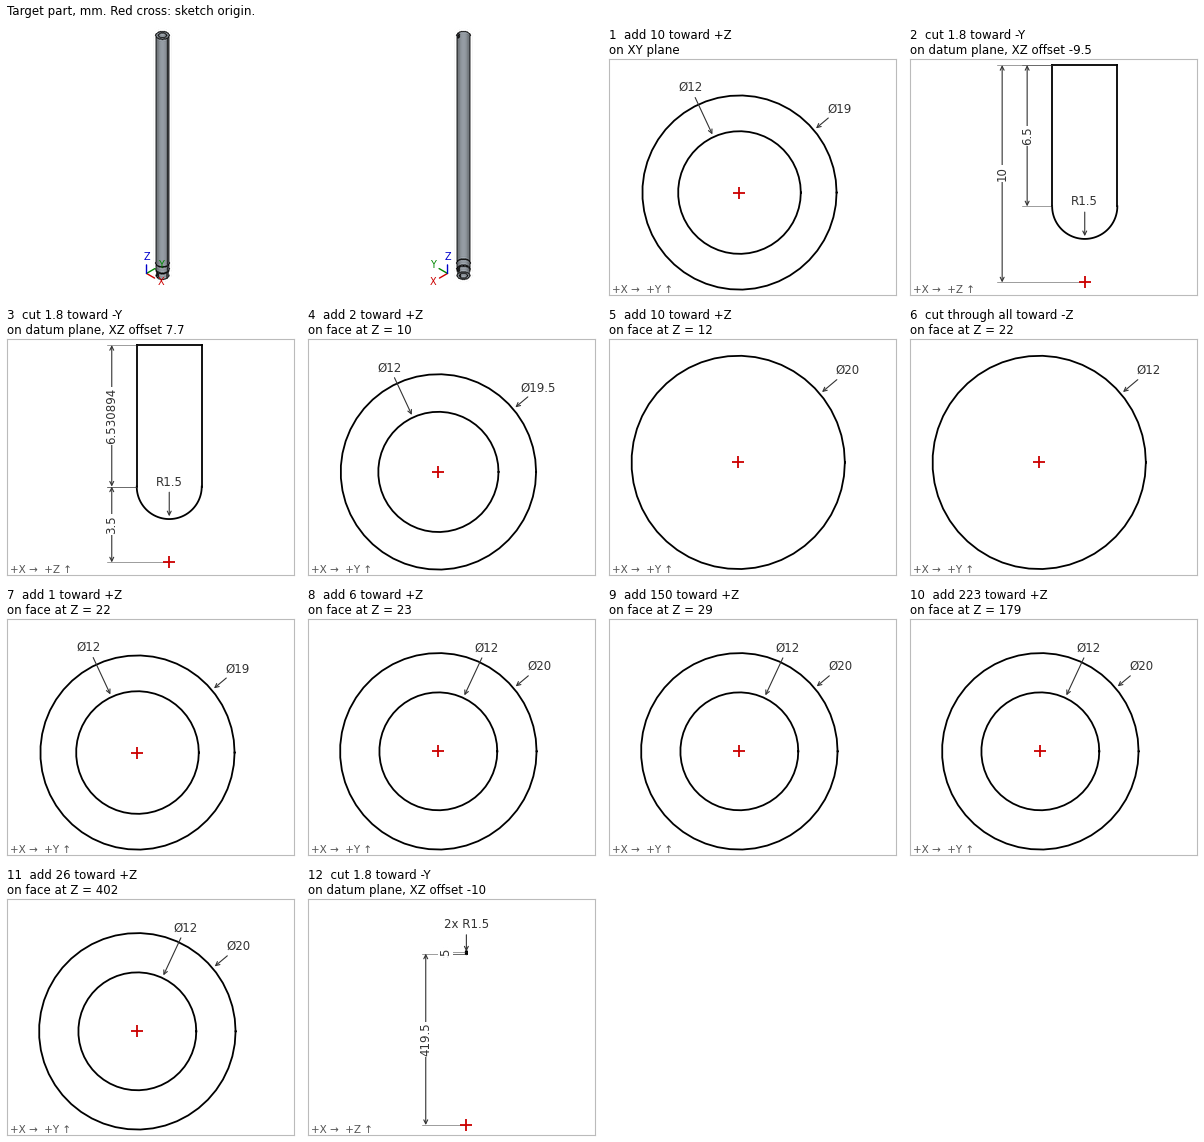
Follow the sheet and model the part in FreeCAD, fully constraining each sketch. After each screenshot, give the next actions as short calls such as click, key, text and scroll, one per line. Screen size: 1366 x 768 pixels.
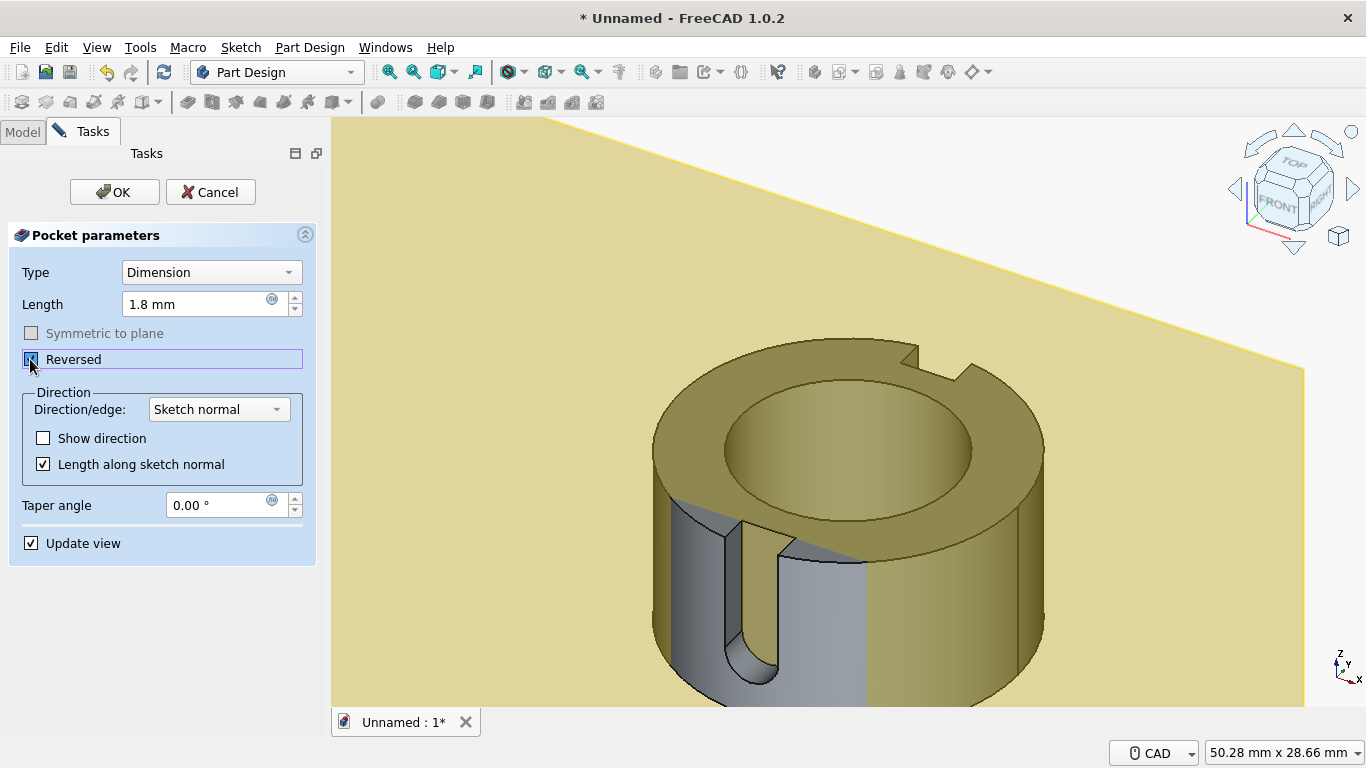
click(115, 192)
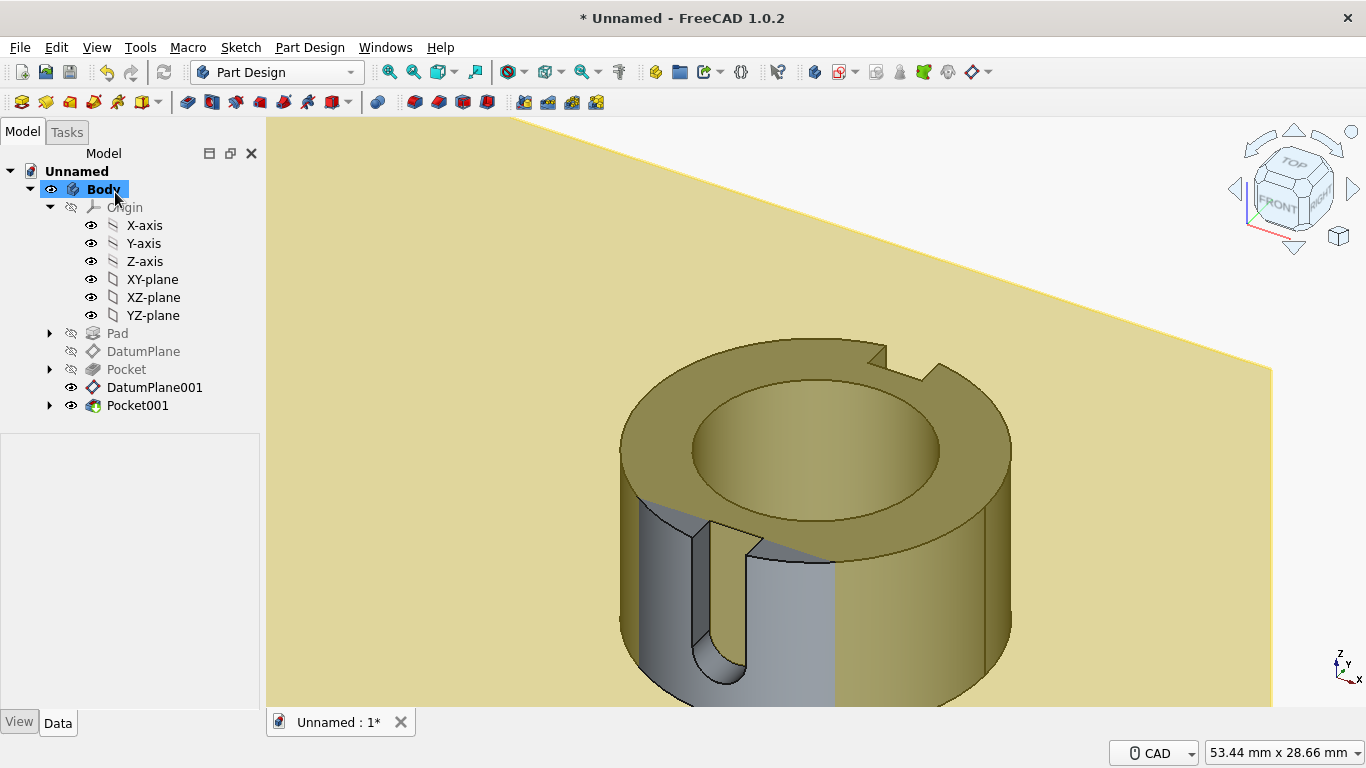
click(116, 387)
key(space)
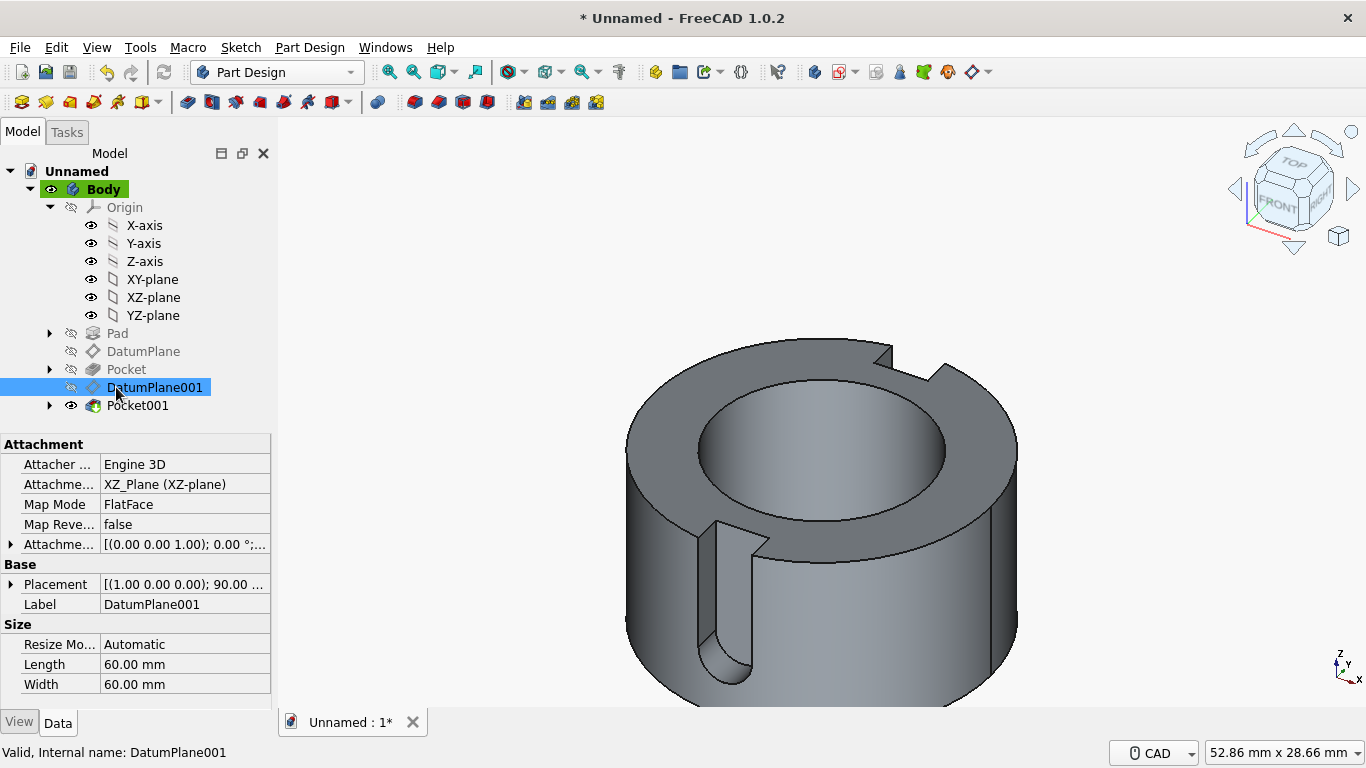
click(390, 72)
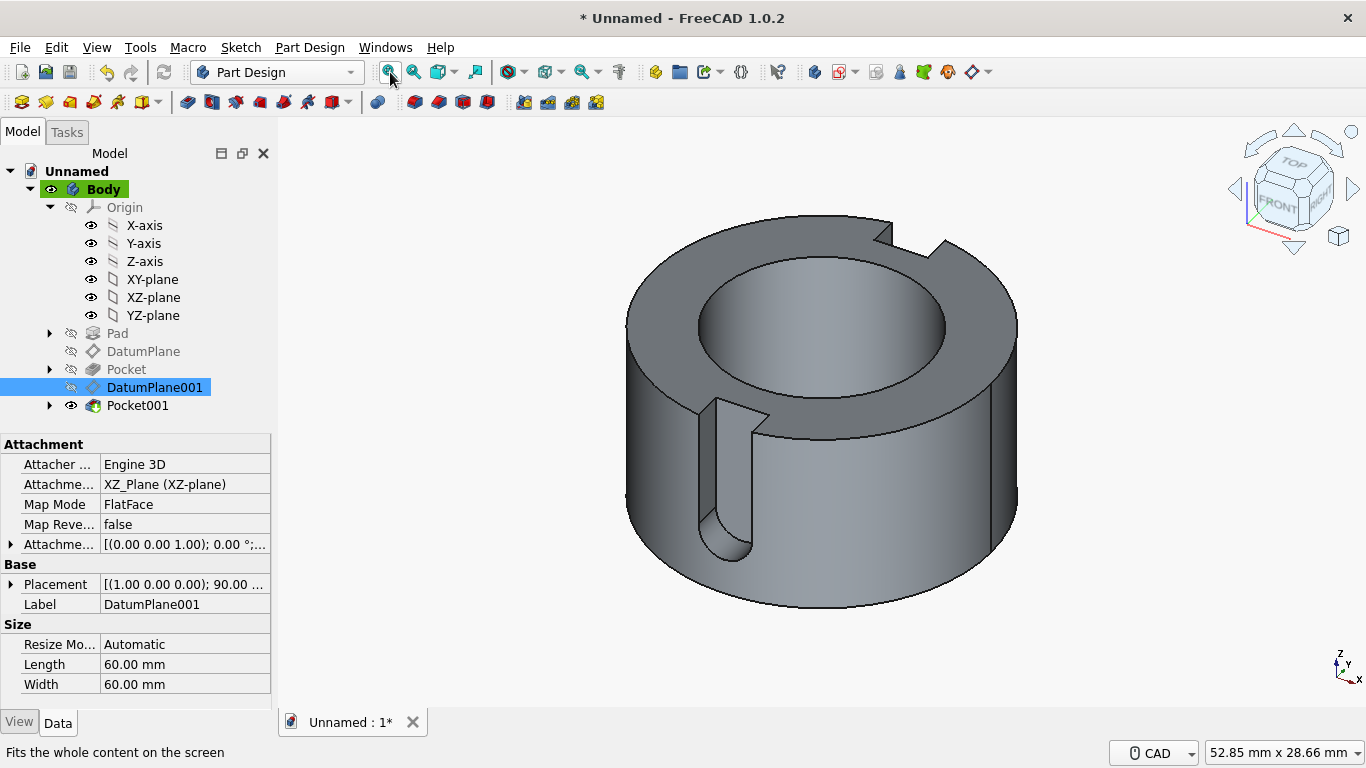
click(780, 240)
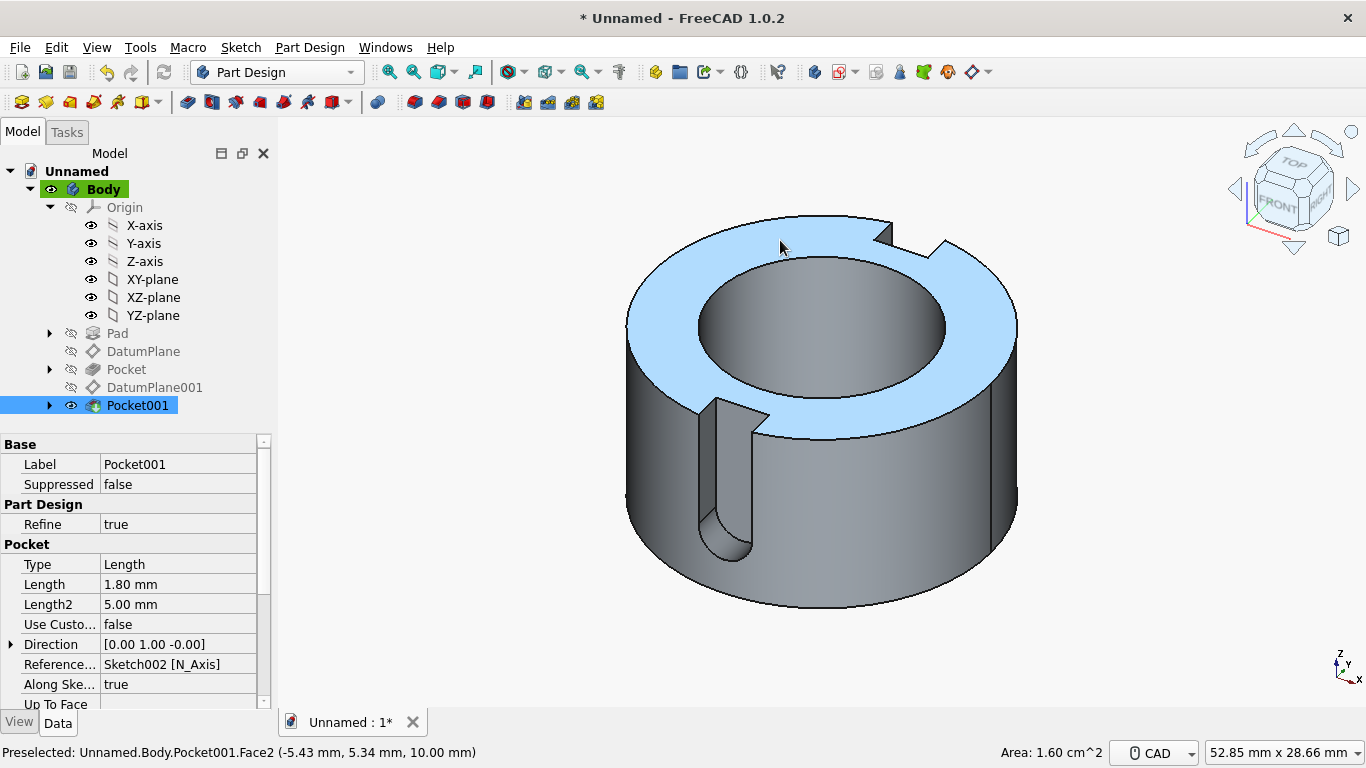
click(840, 72)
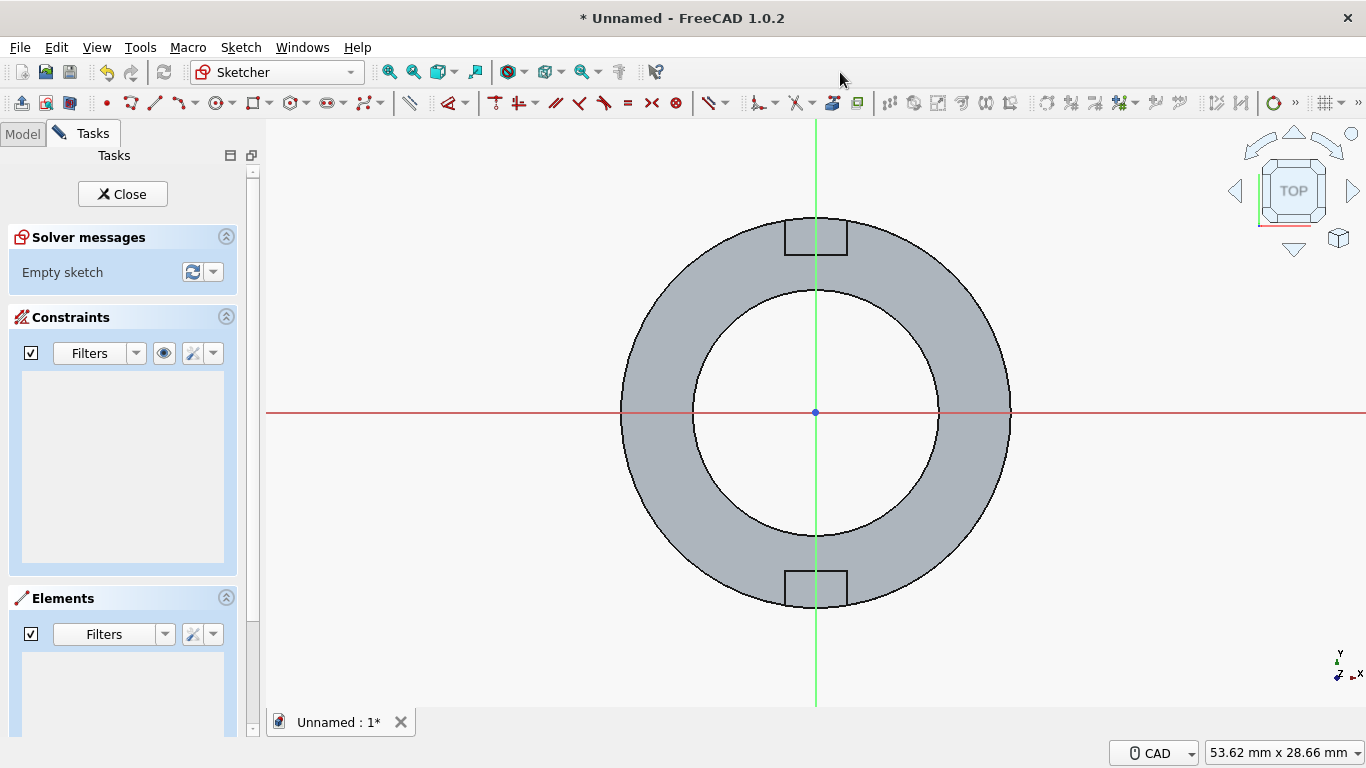
click(216, 104)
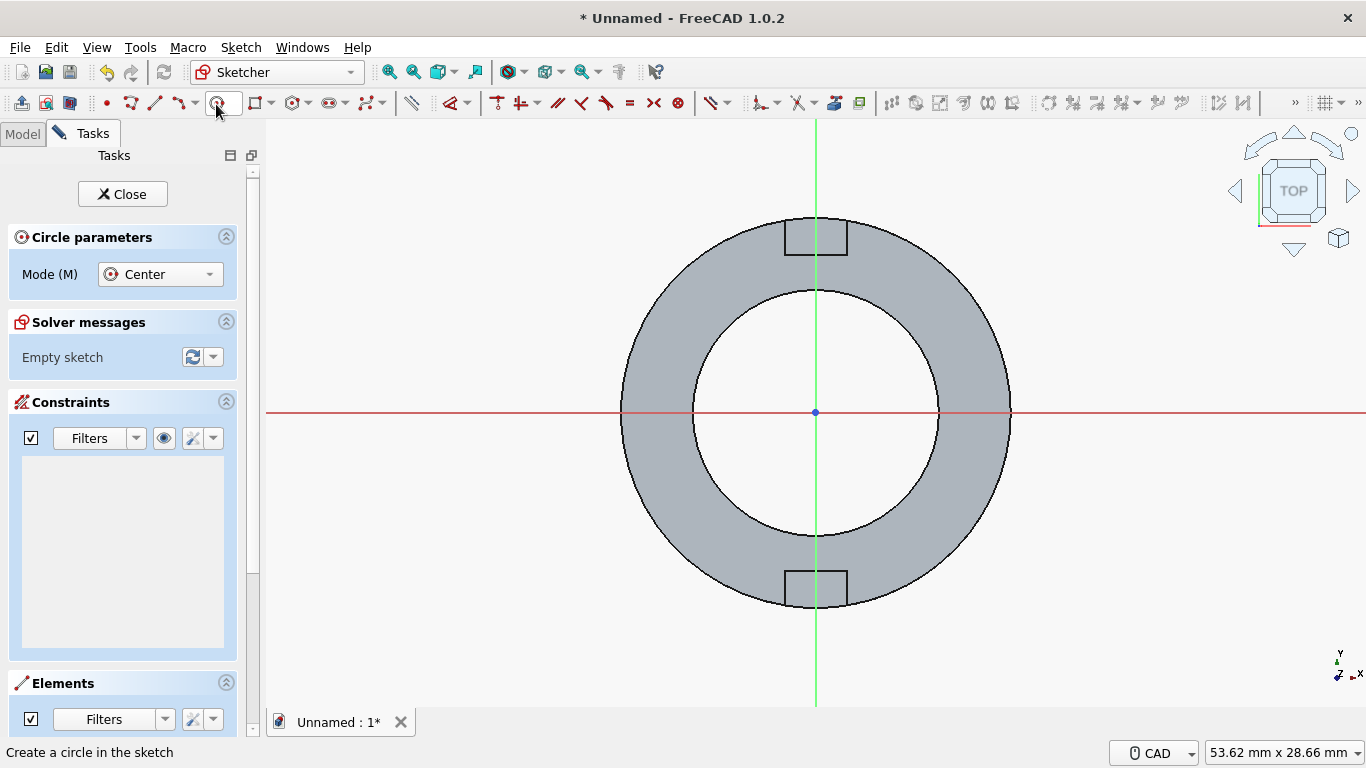
click(816, 413)
click(957, 272)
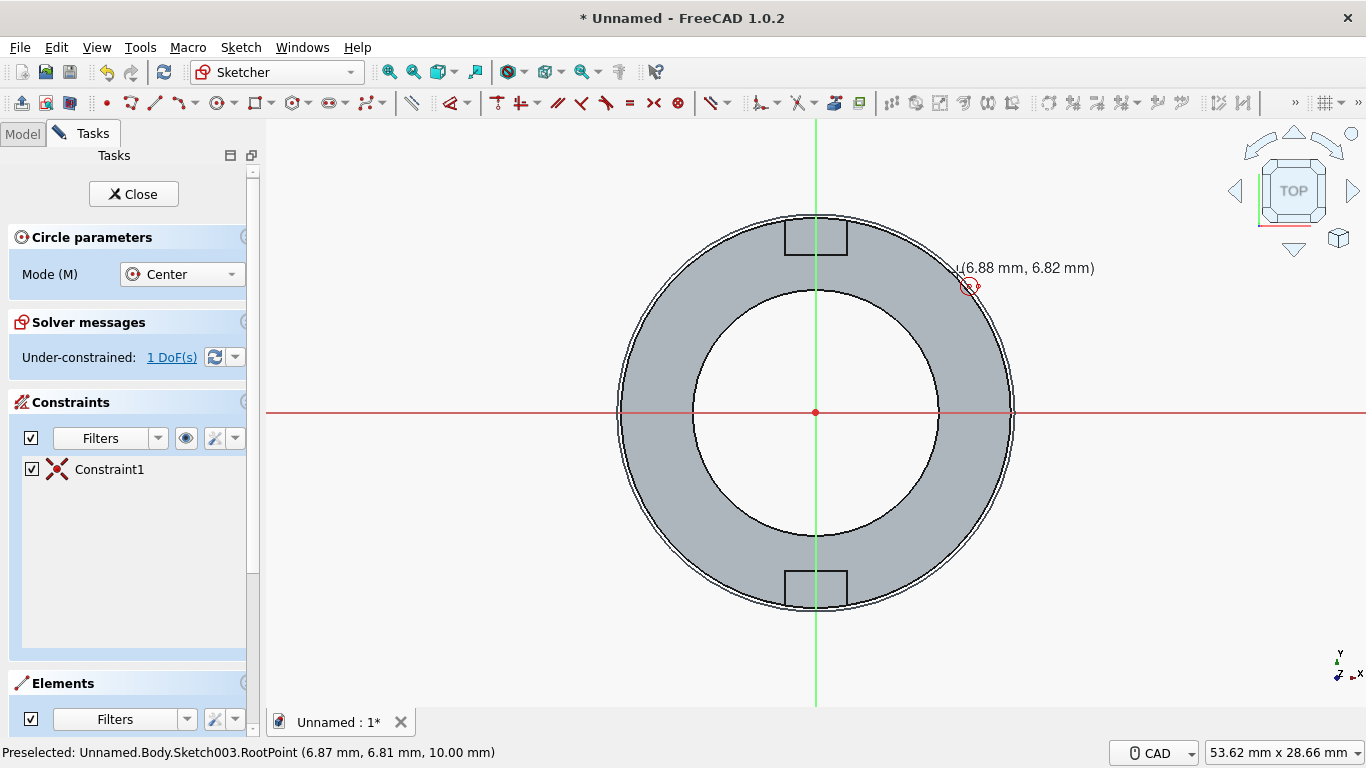
click(816, 413)
click(903, 326)
key(Escape)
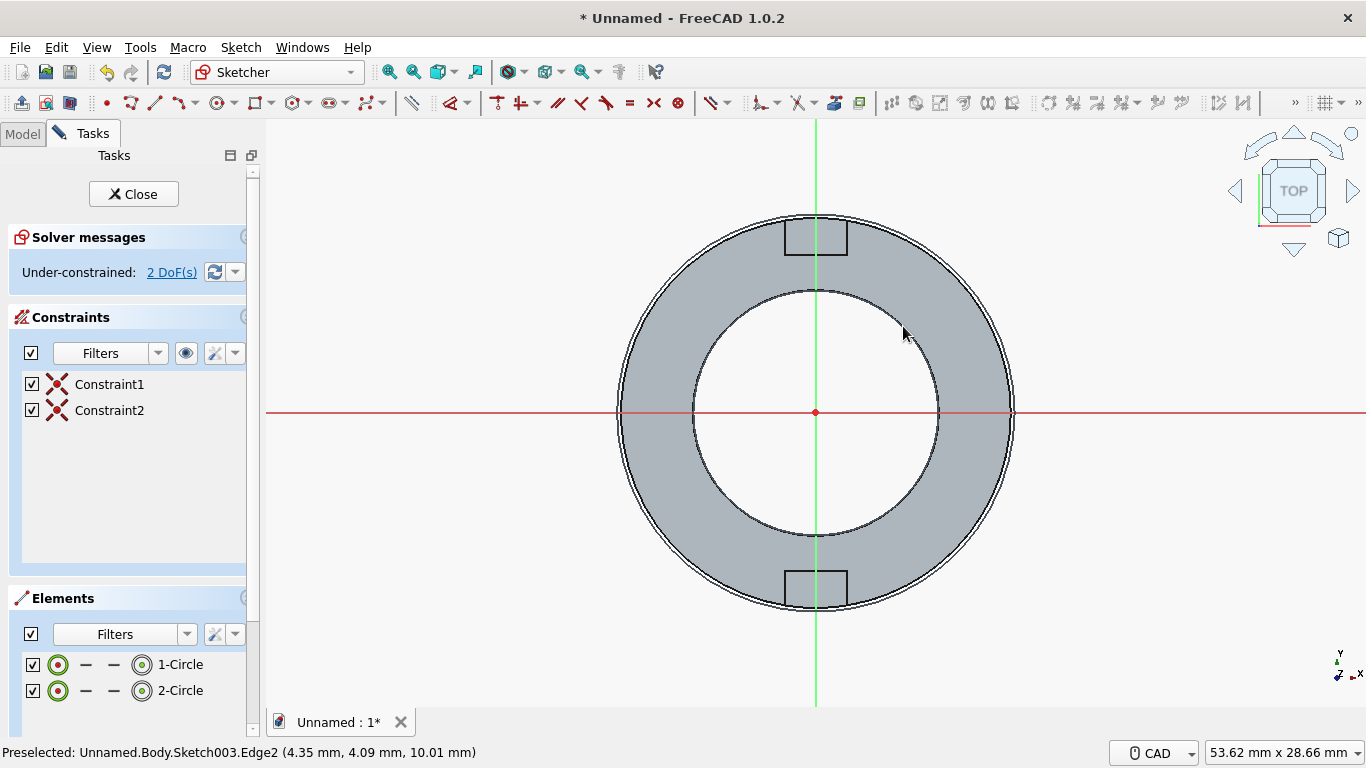
click(450, 104)